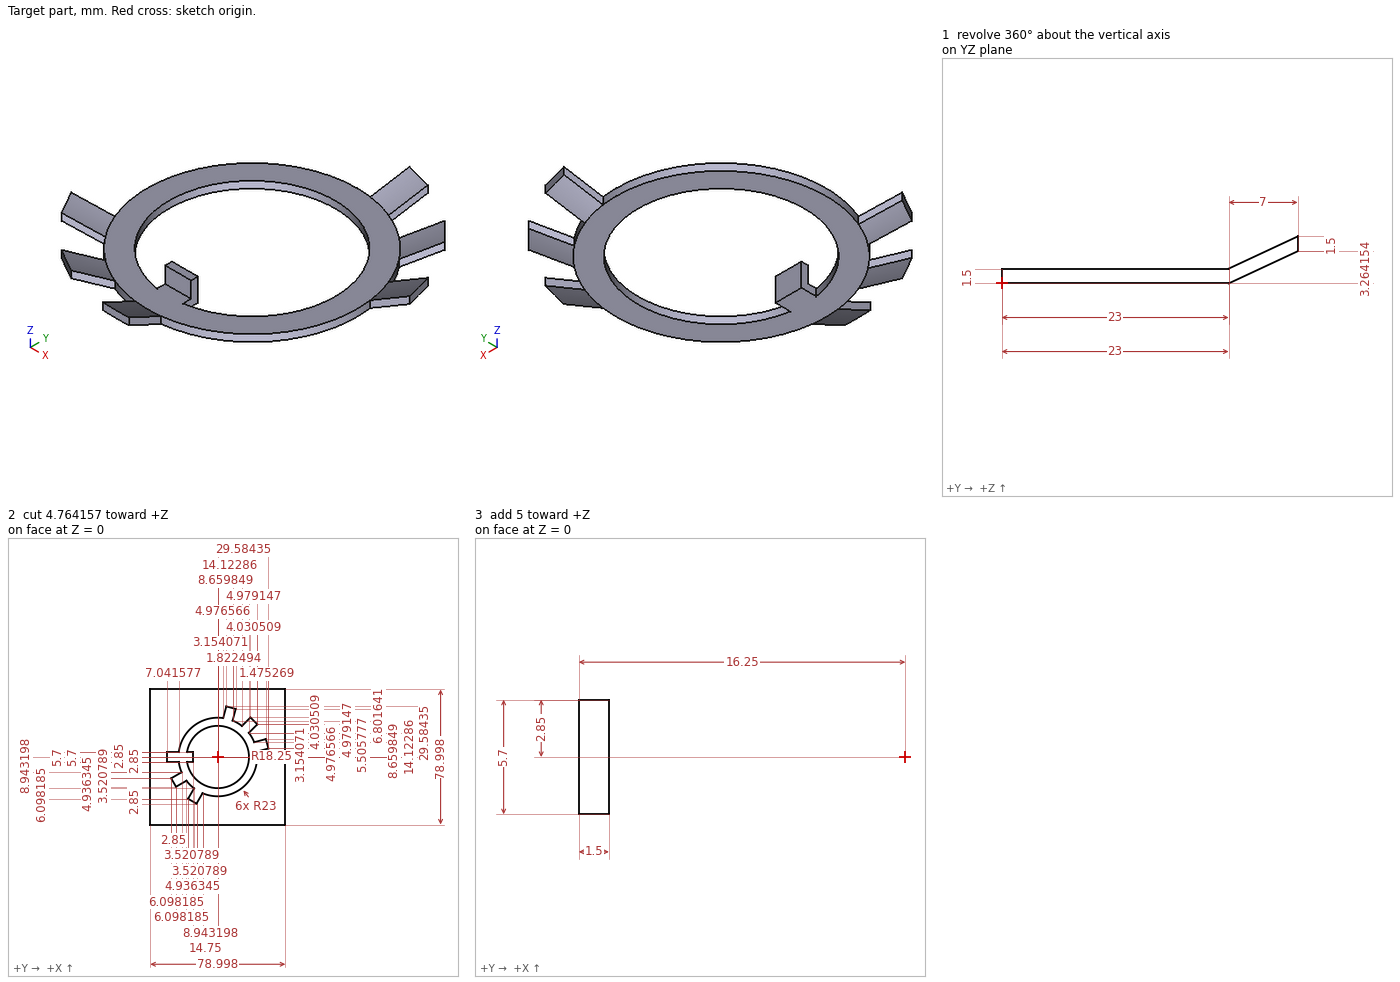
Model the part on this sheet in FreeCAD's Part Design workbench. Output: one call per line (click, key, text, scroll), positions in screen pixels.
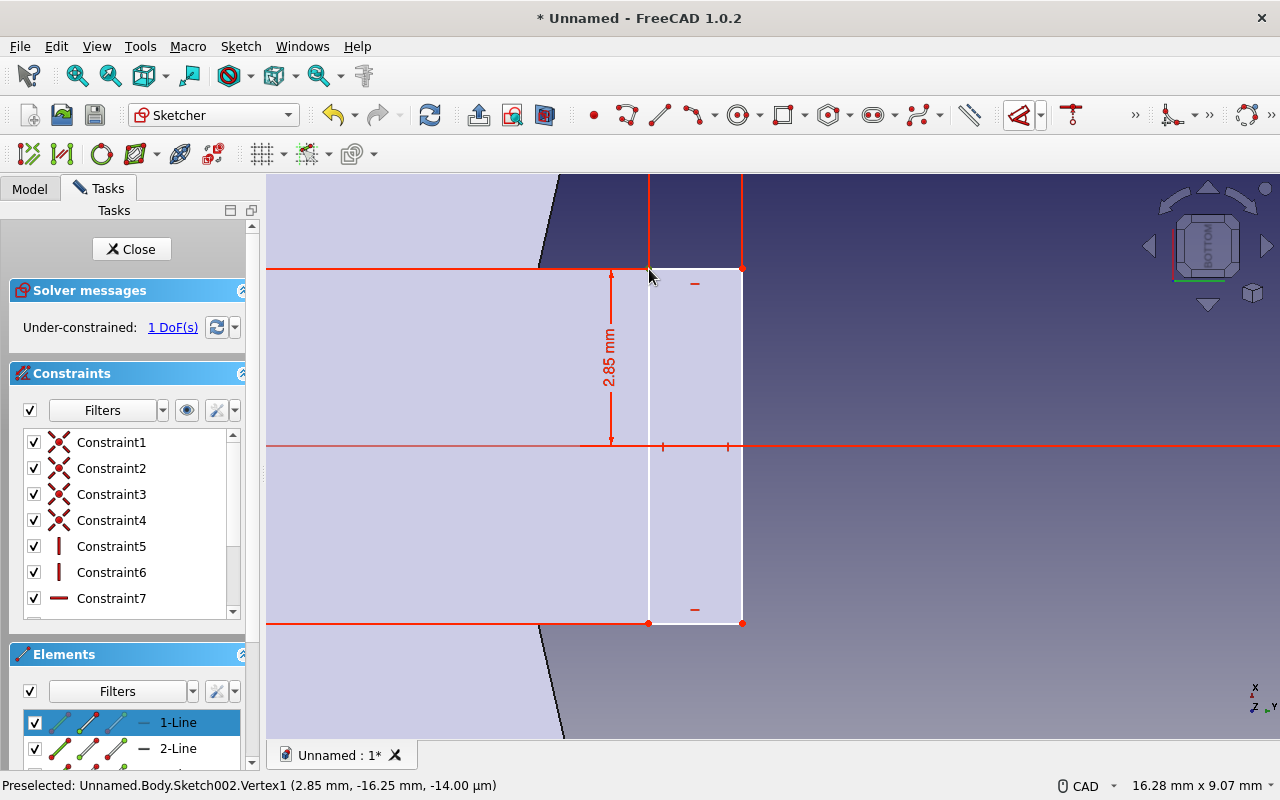
key(l)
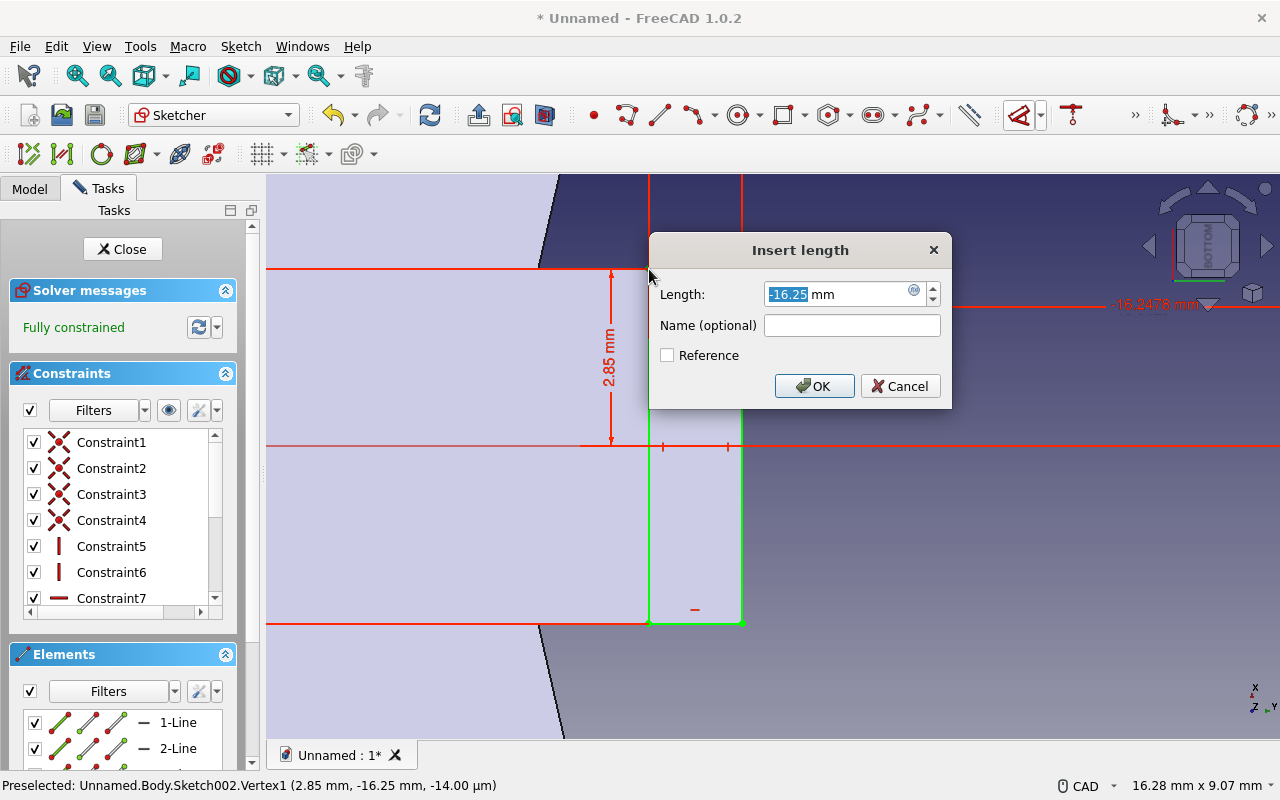
text(-16.25)
key(Return)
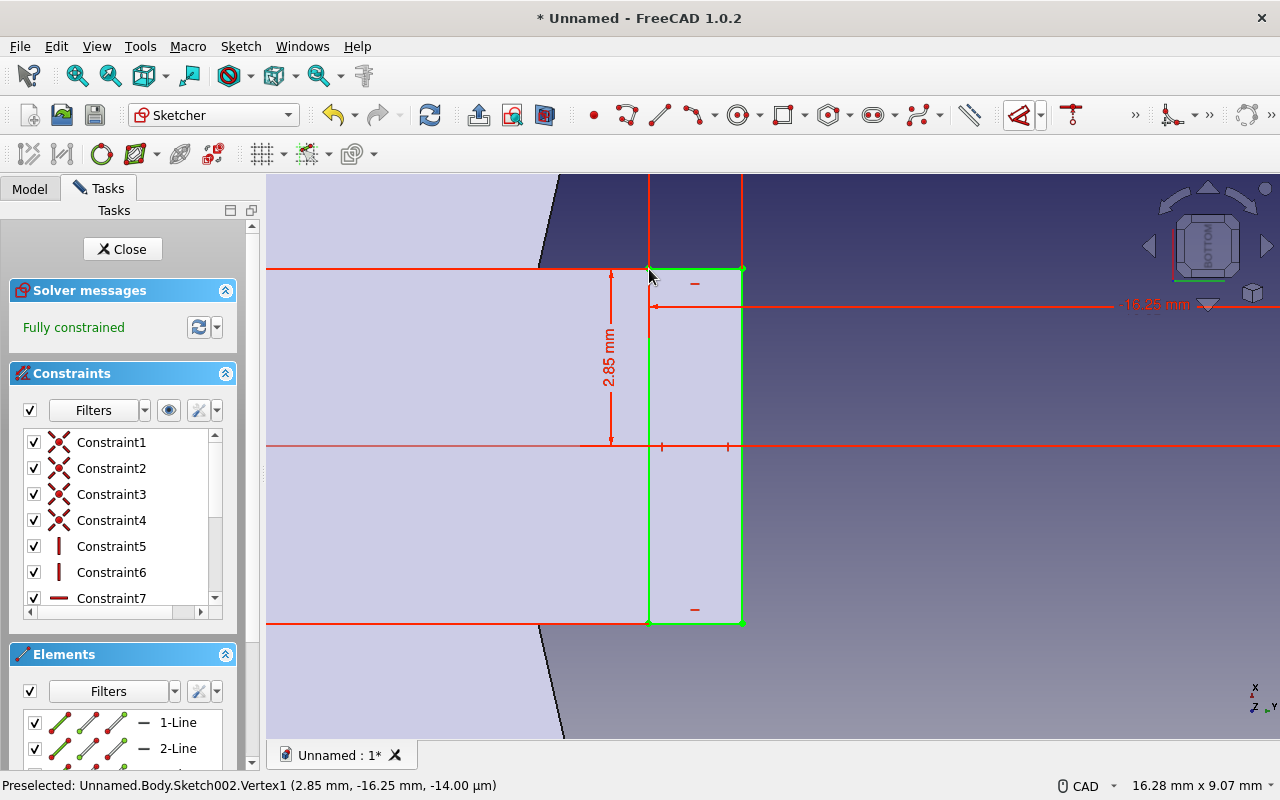
click(123, 249)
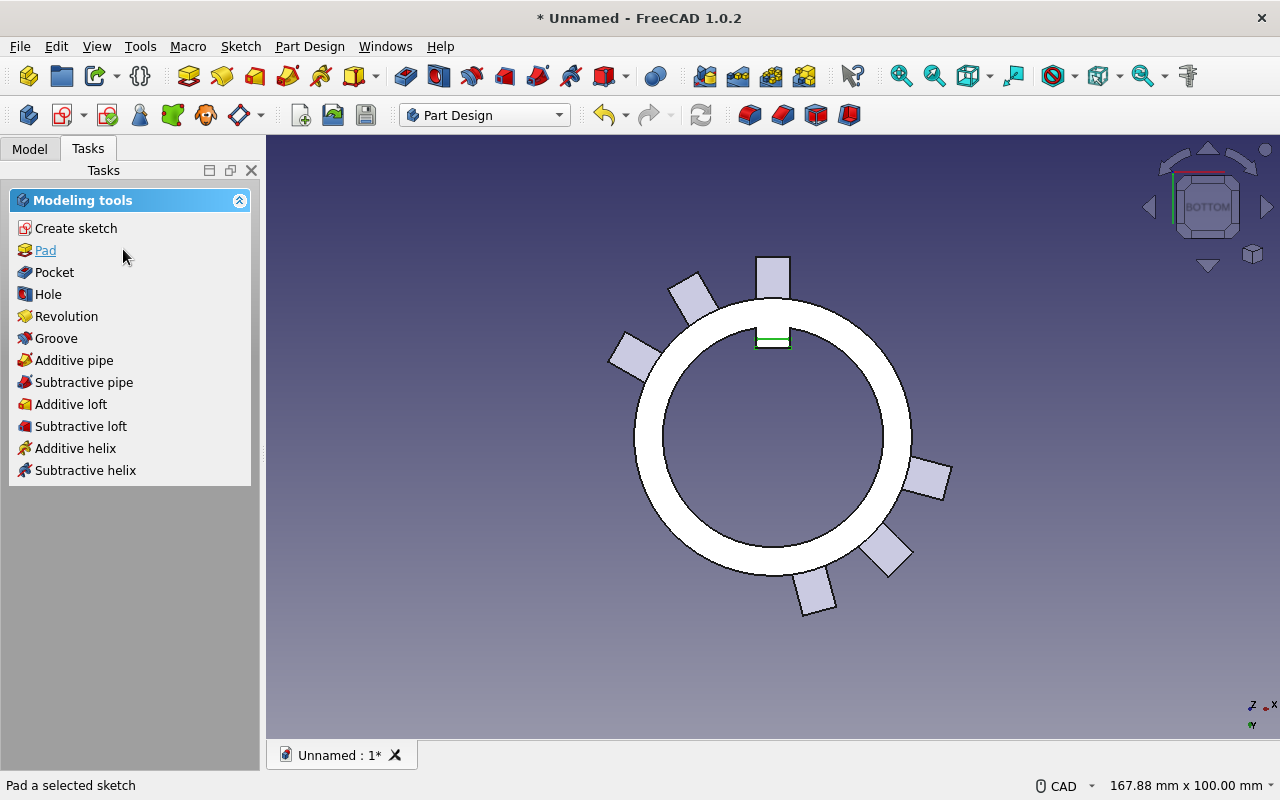
click(189, 76)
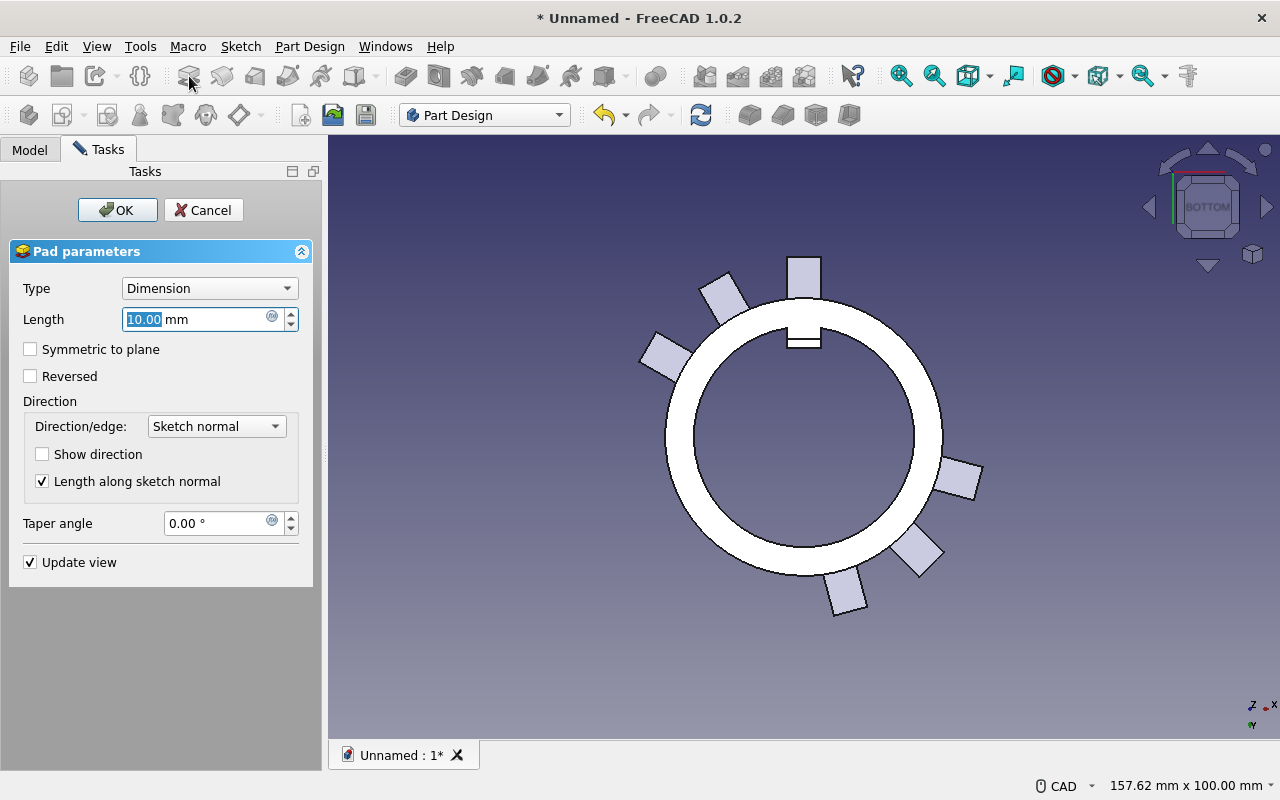
text(5)
key(Tab)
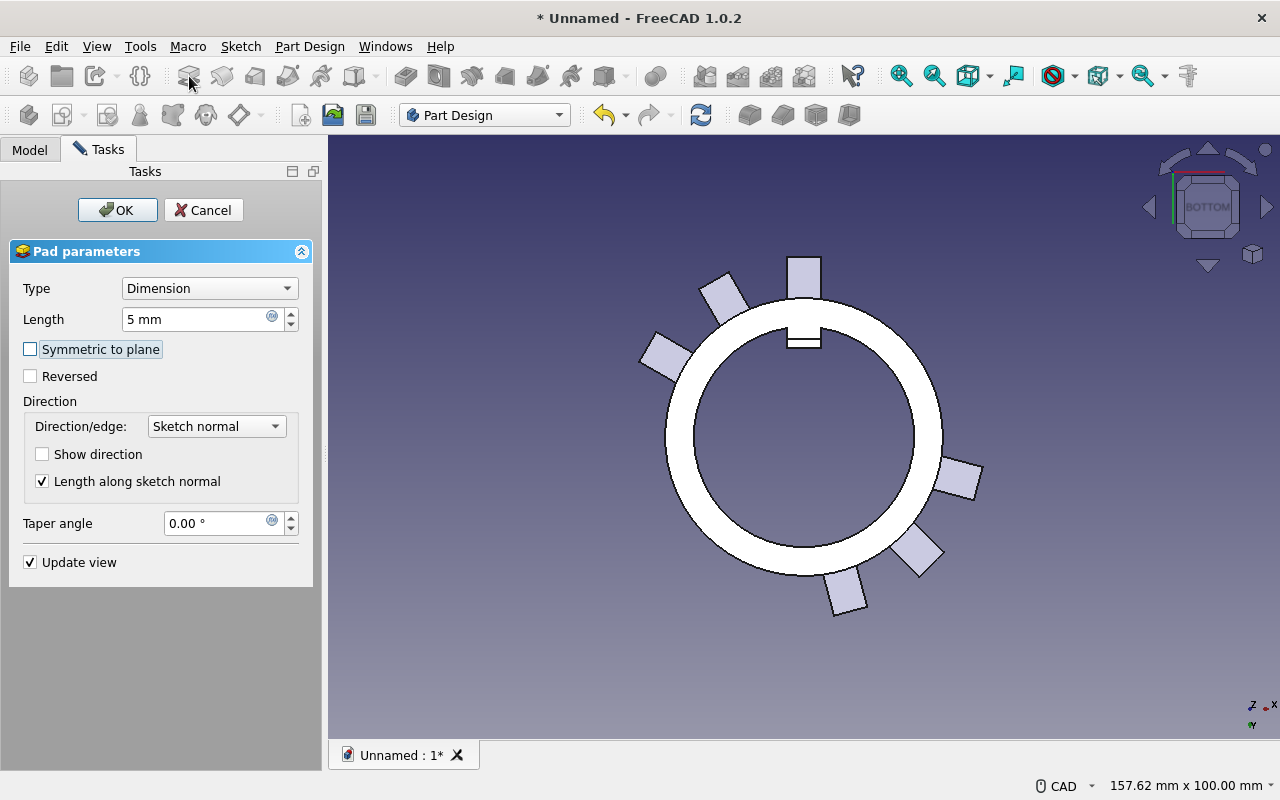
click(31, 376)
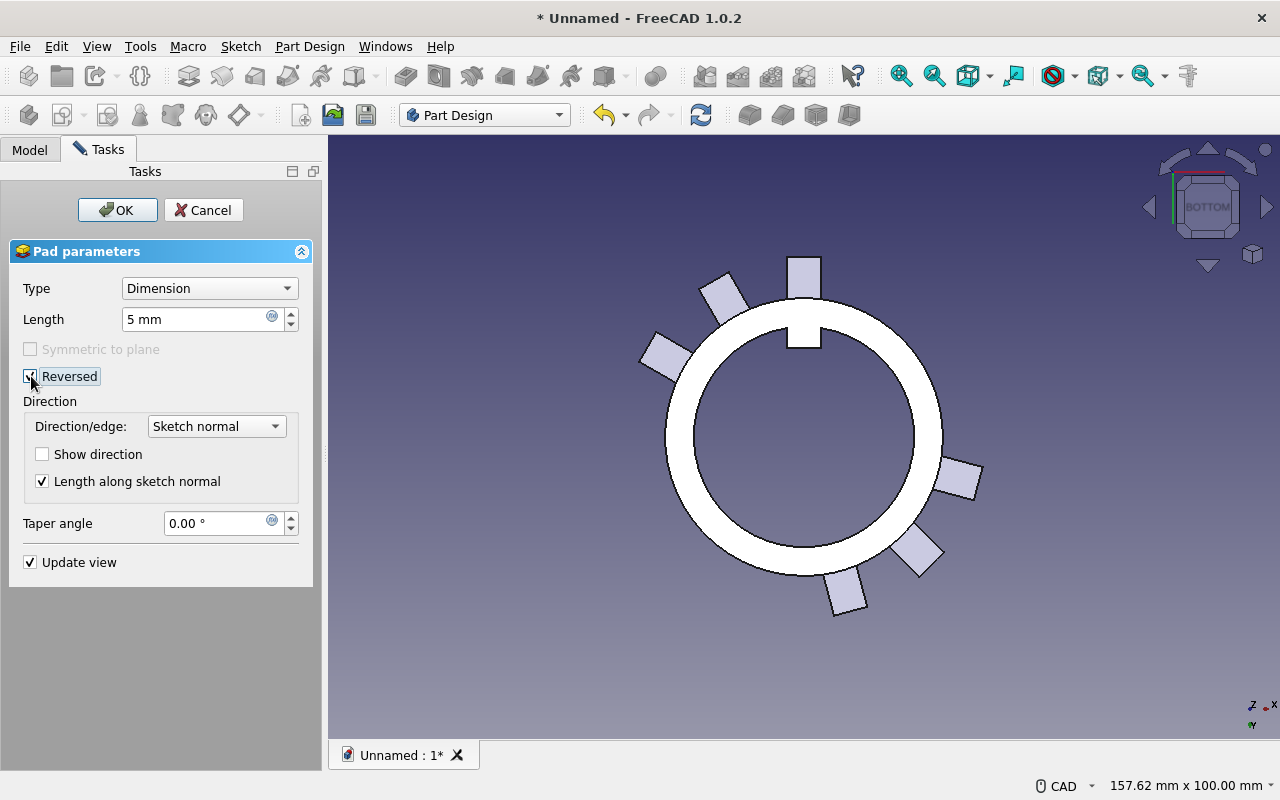
click(118, 210)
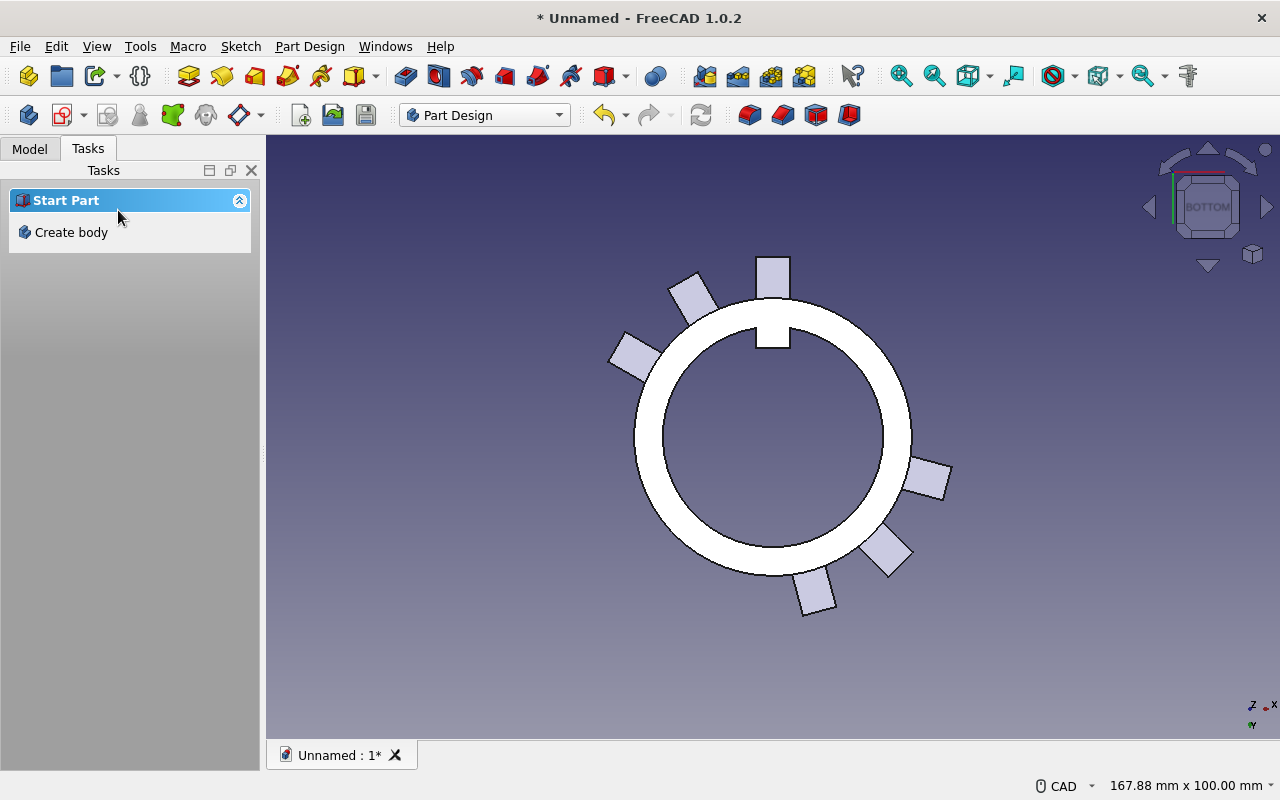
key(0)